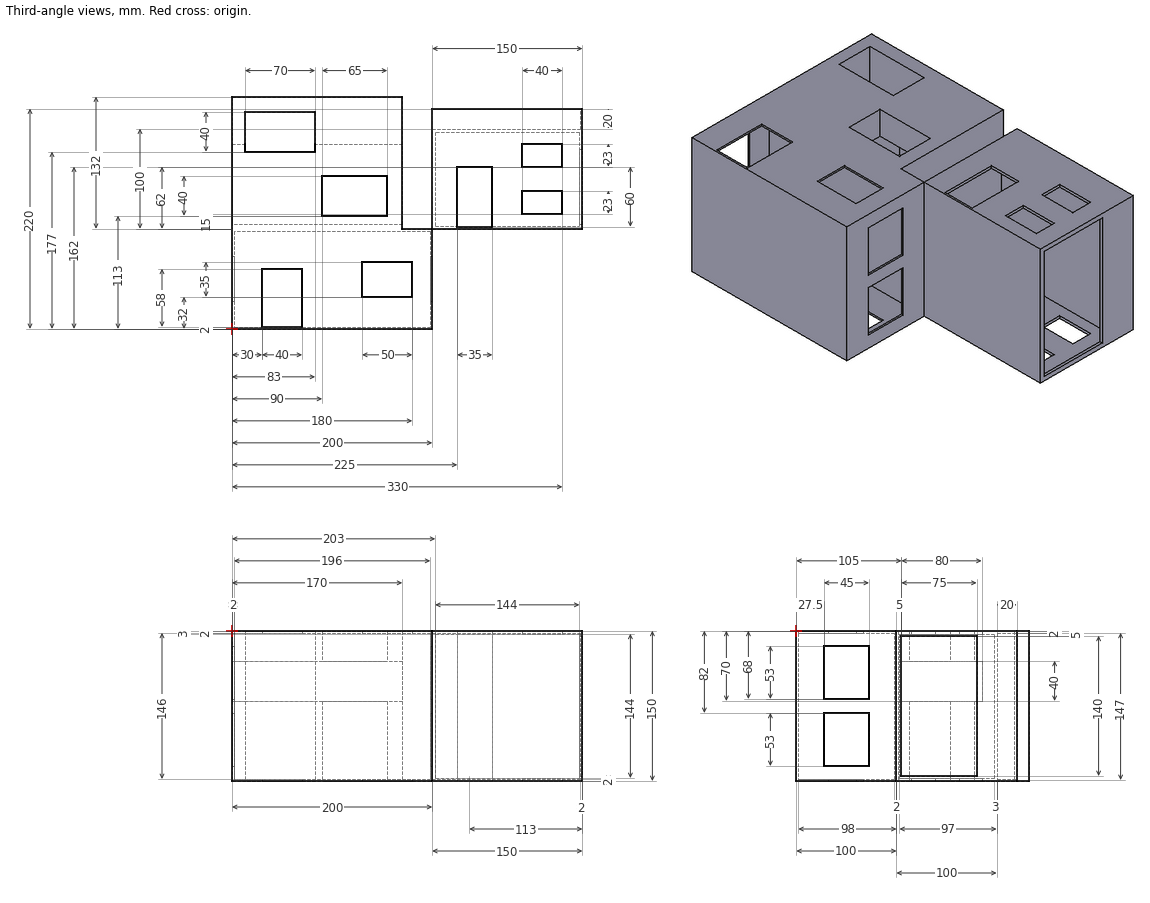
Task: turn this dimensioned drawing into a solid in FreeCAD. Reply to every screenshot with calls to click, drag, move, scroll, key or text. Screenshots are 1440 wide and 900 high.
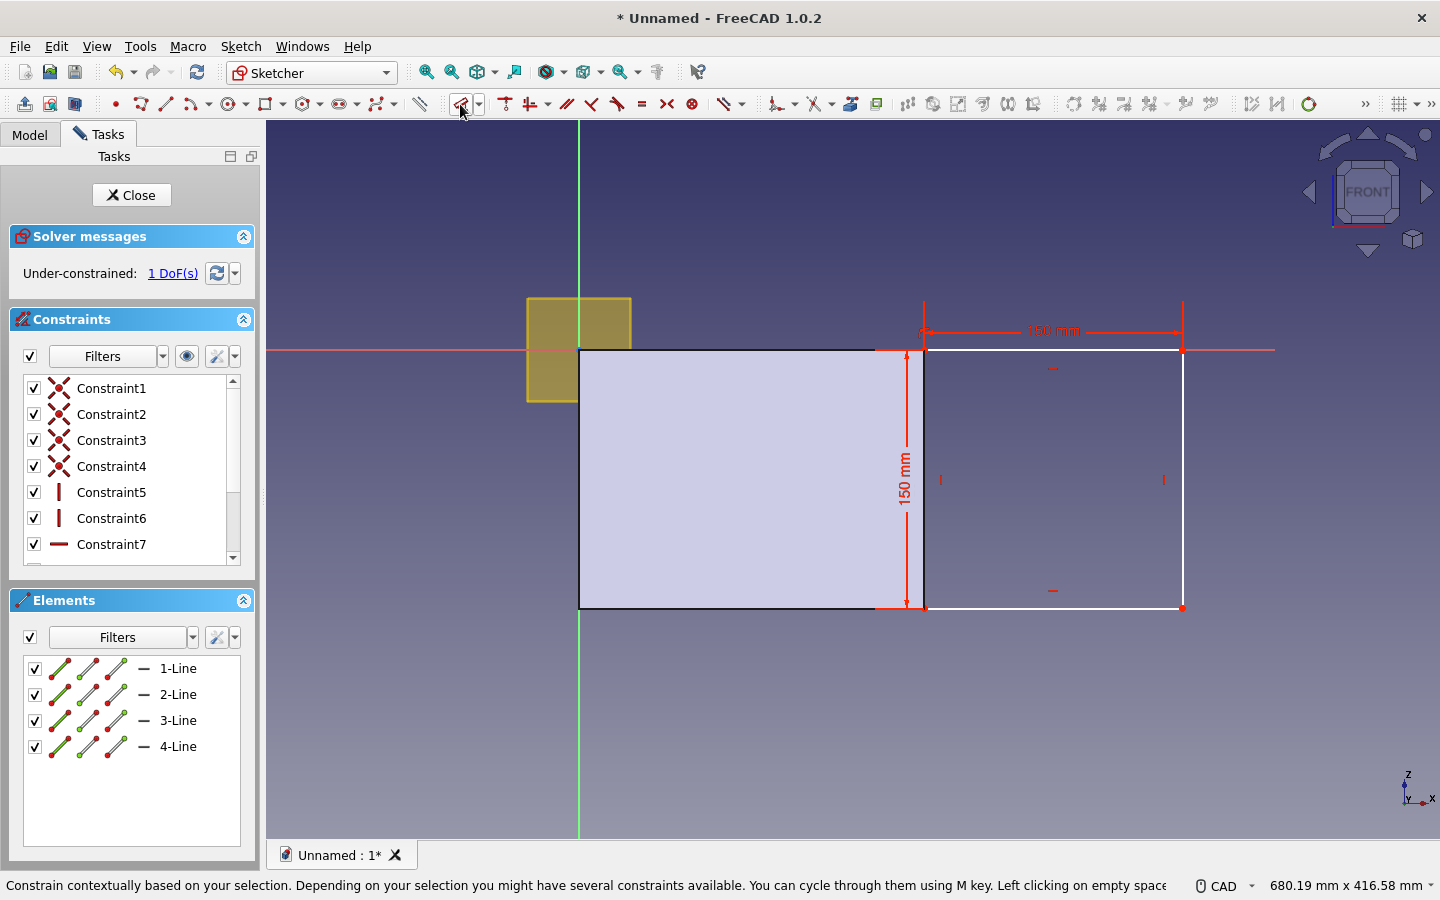
click(924, 350)
click(752, 316)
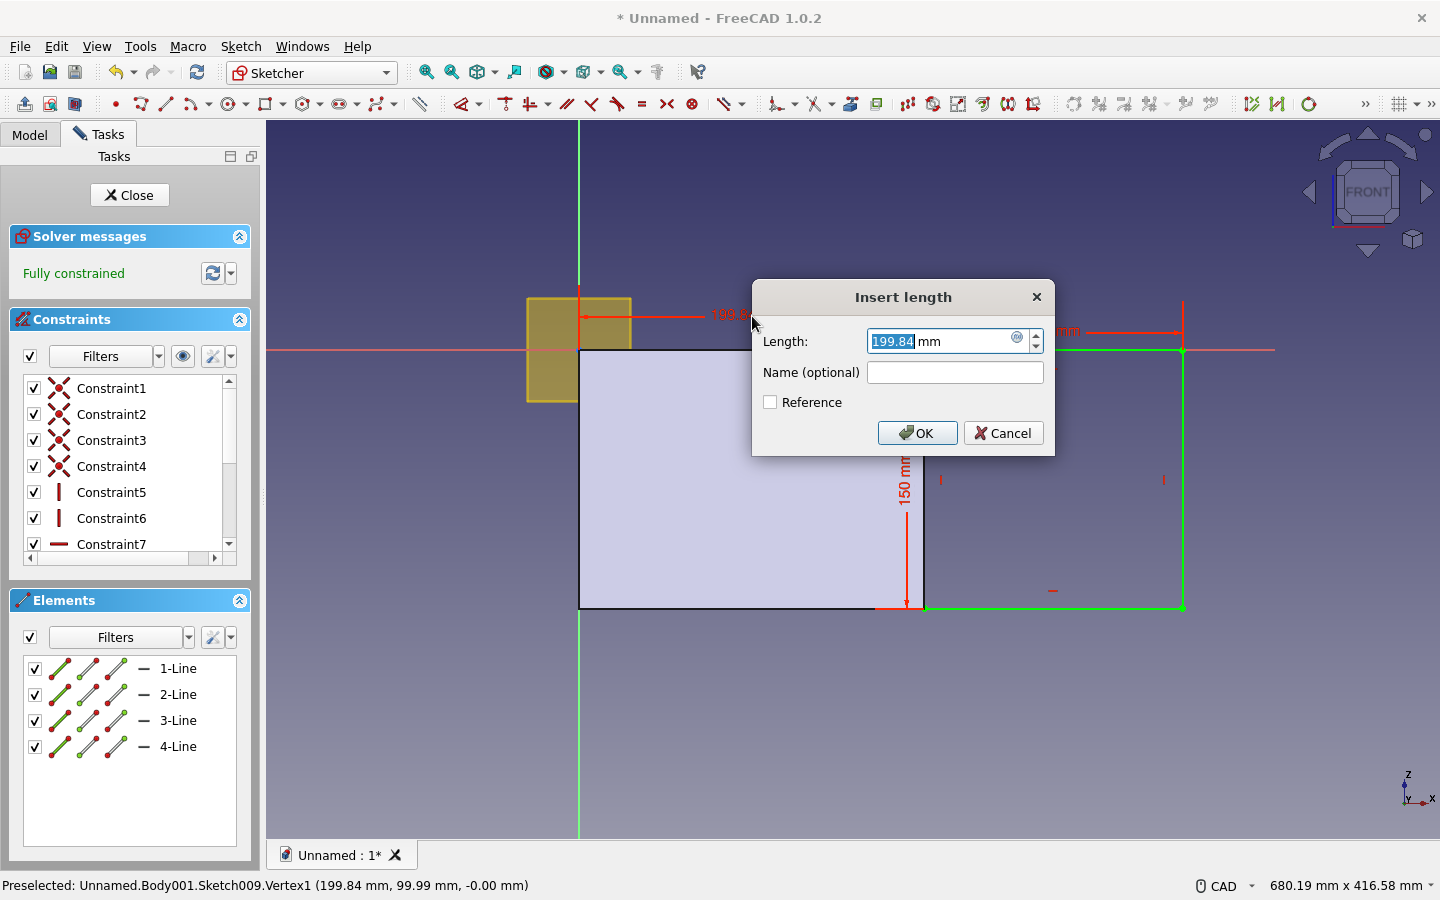
text(200)
key(Return)
key(Escape)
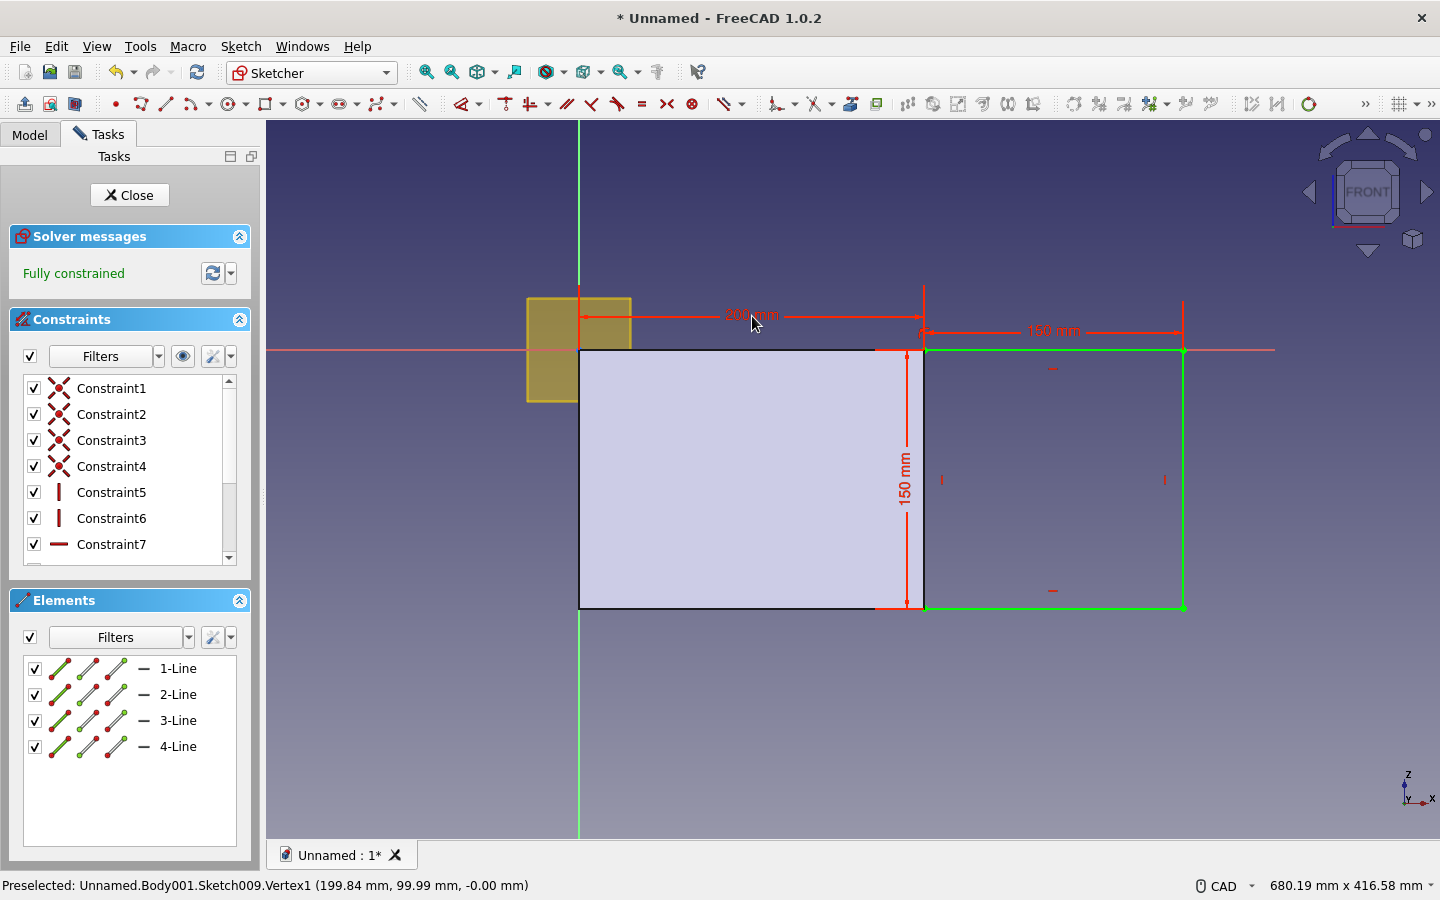
click(130, 195)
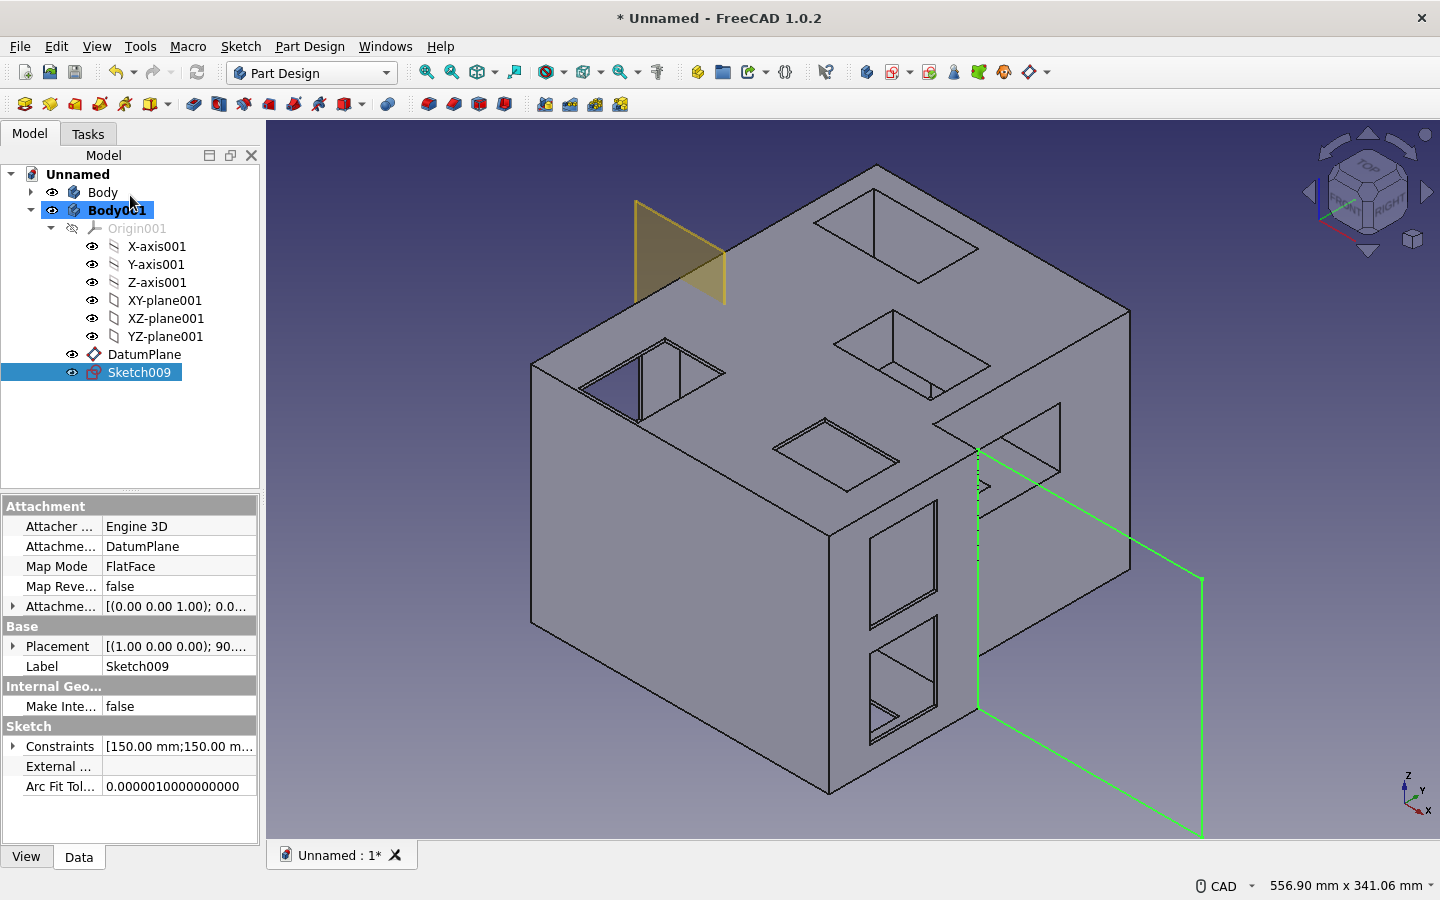
click(25, 104)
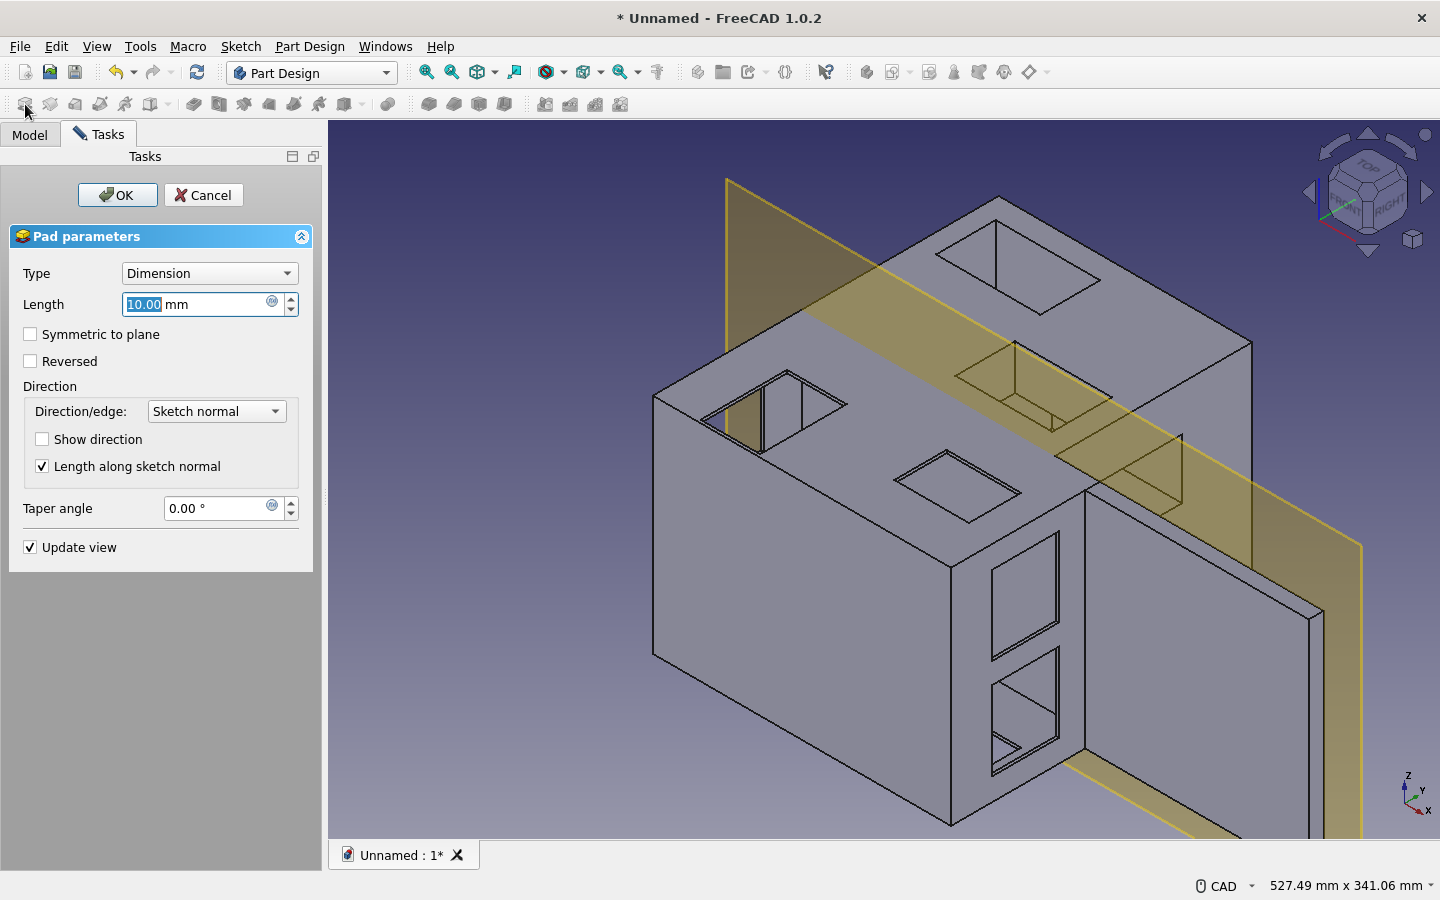
text(100)
key(Tab)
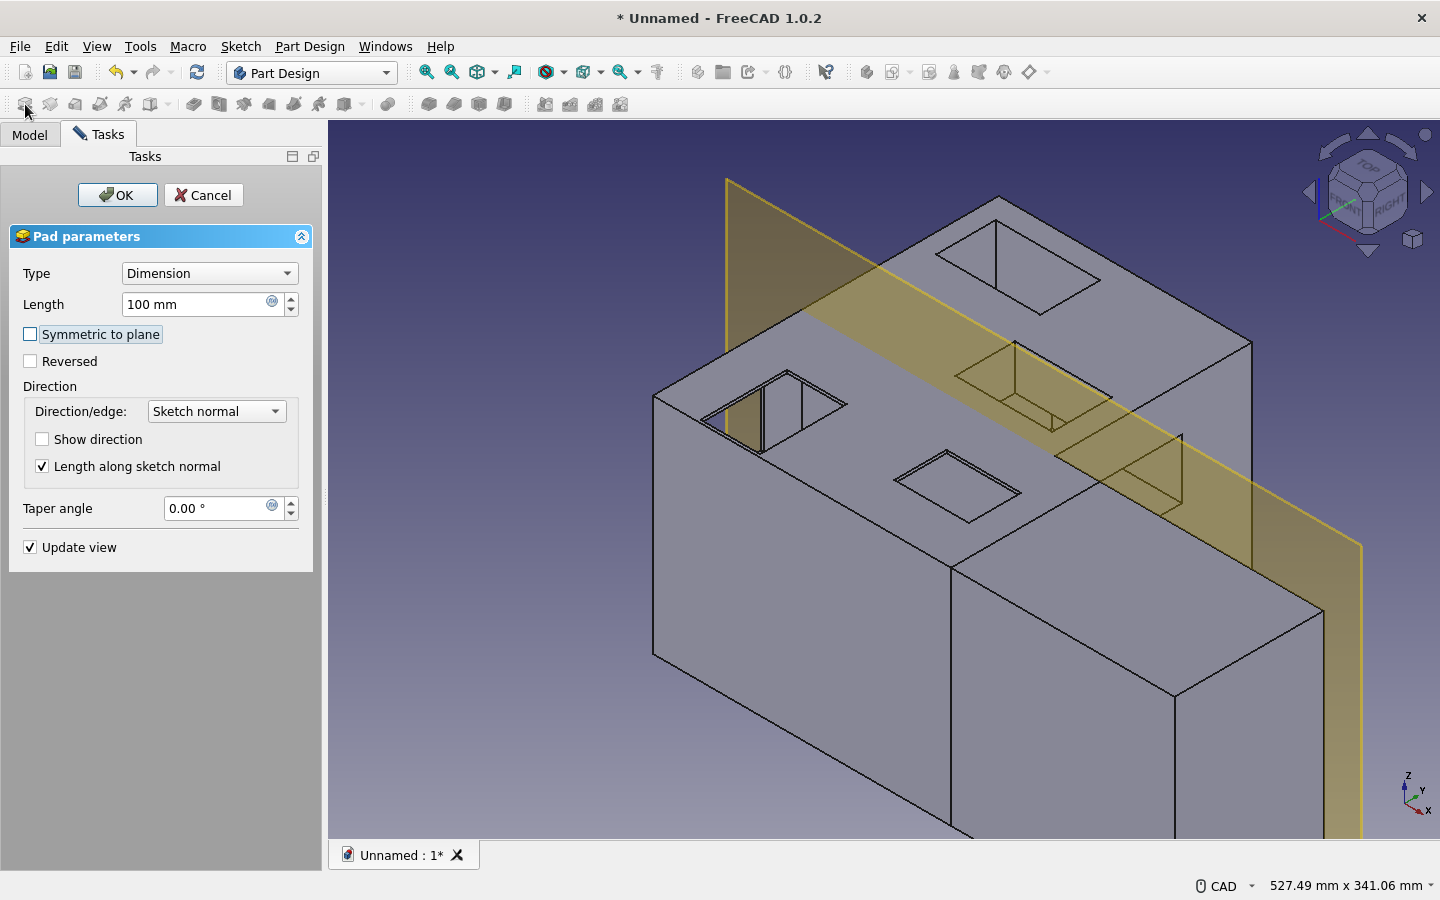
click(31, 361)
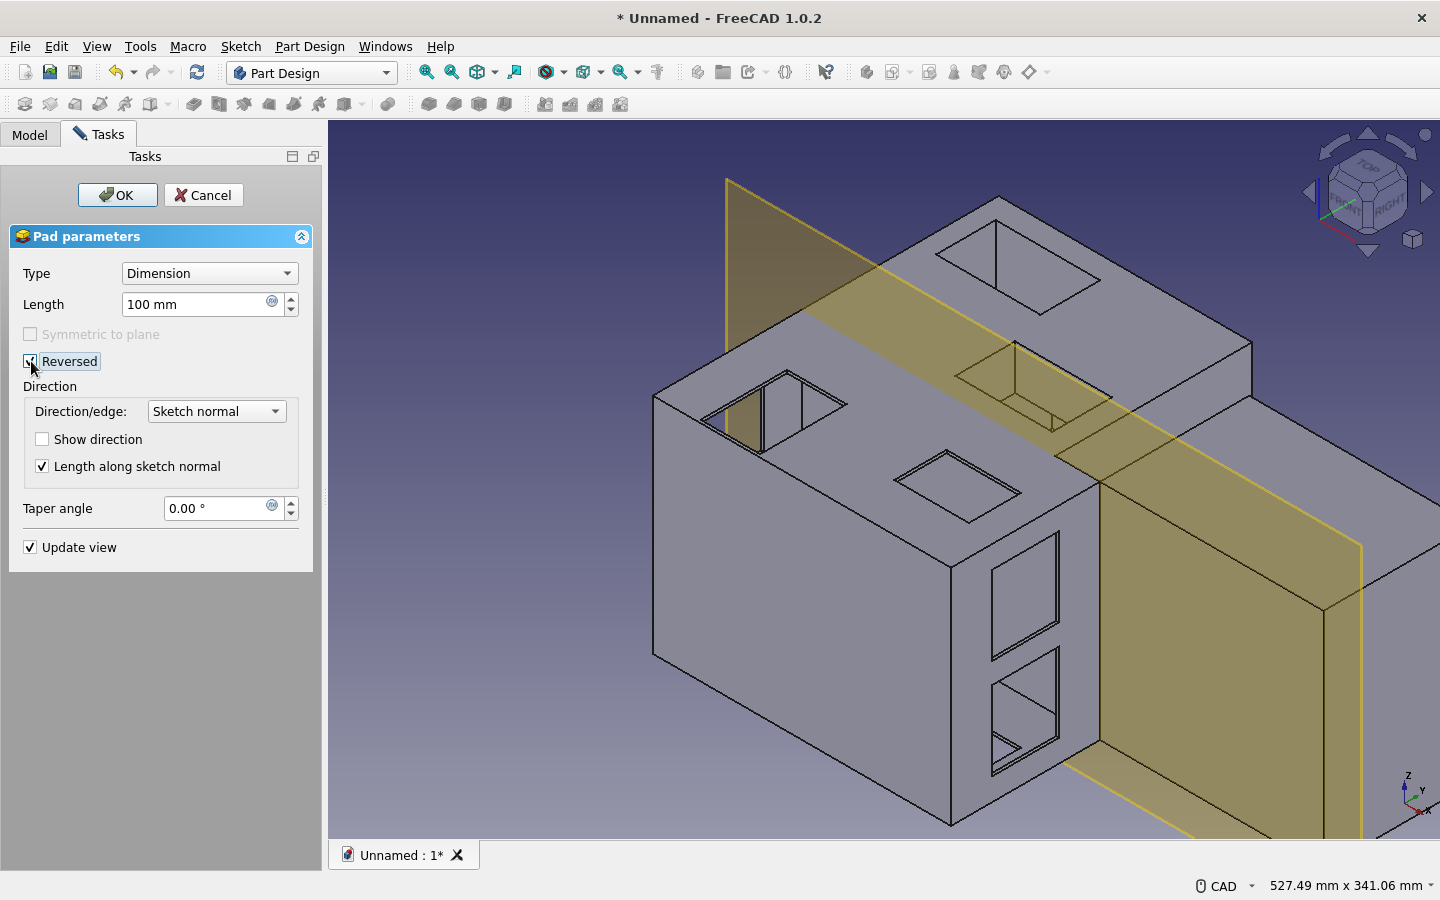
click(118, 195)